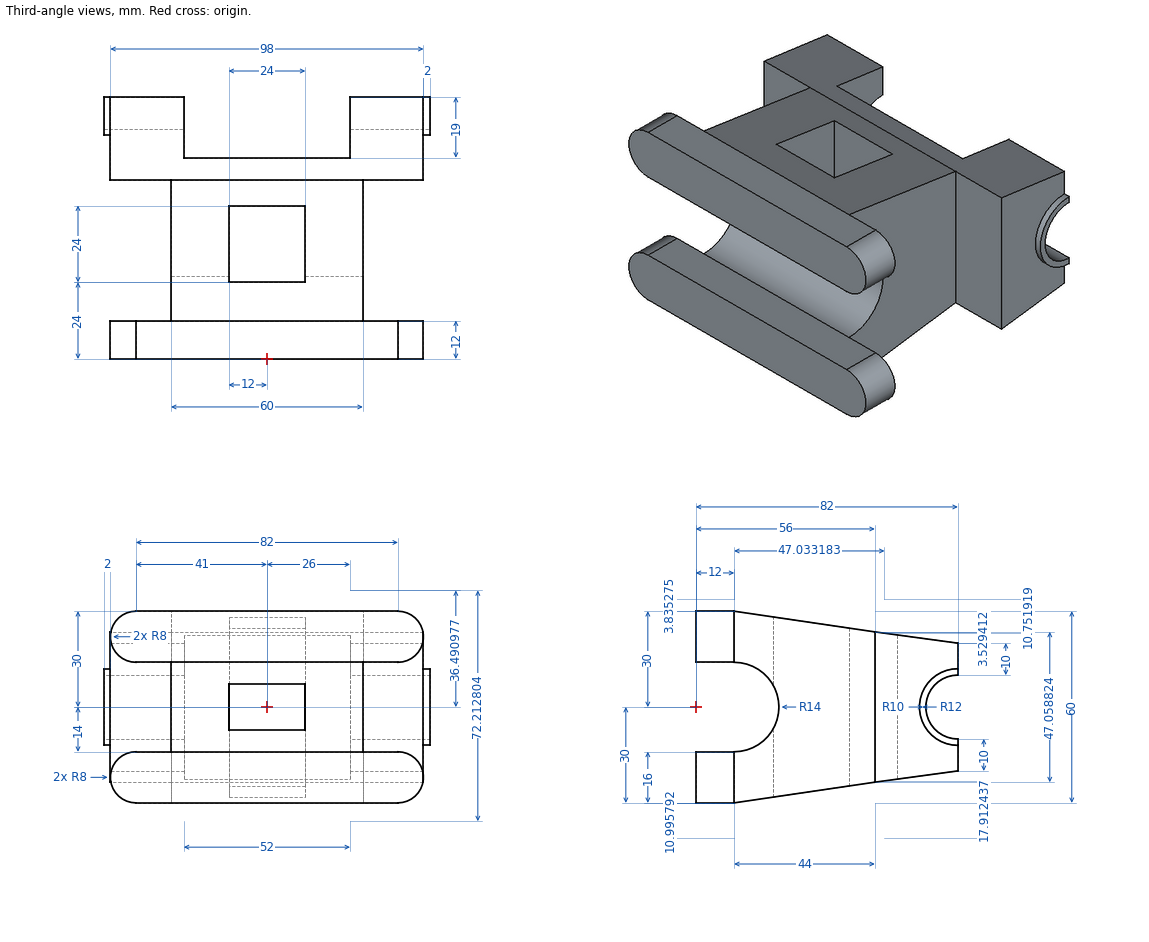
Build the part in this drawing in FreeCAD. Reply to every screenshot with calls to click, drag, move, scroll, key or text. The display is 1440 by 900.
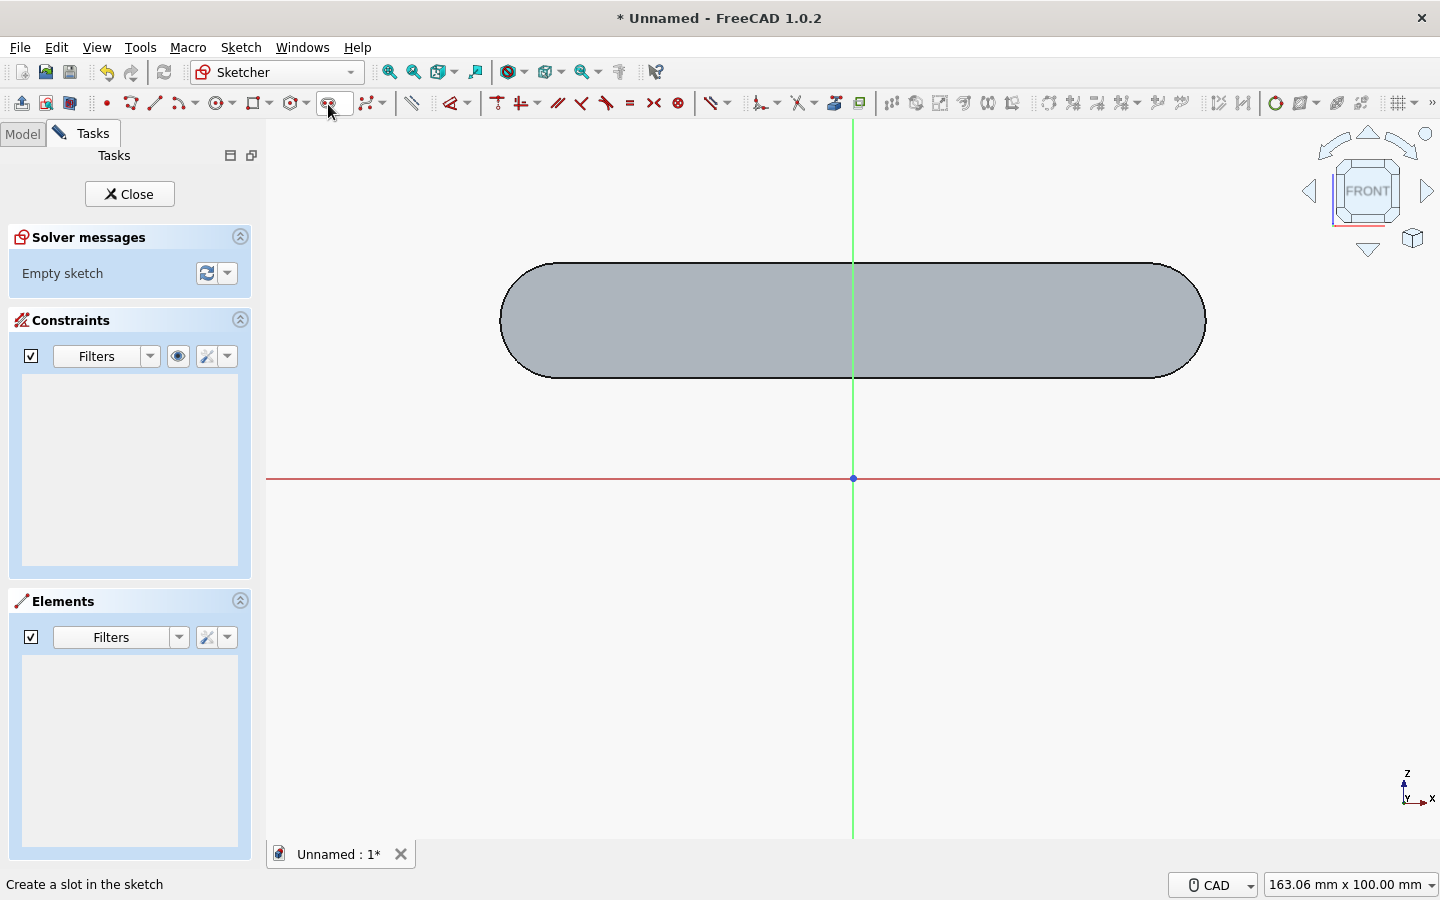
click(558, 637)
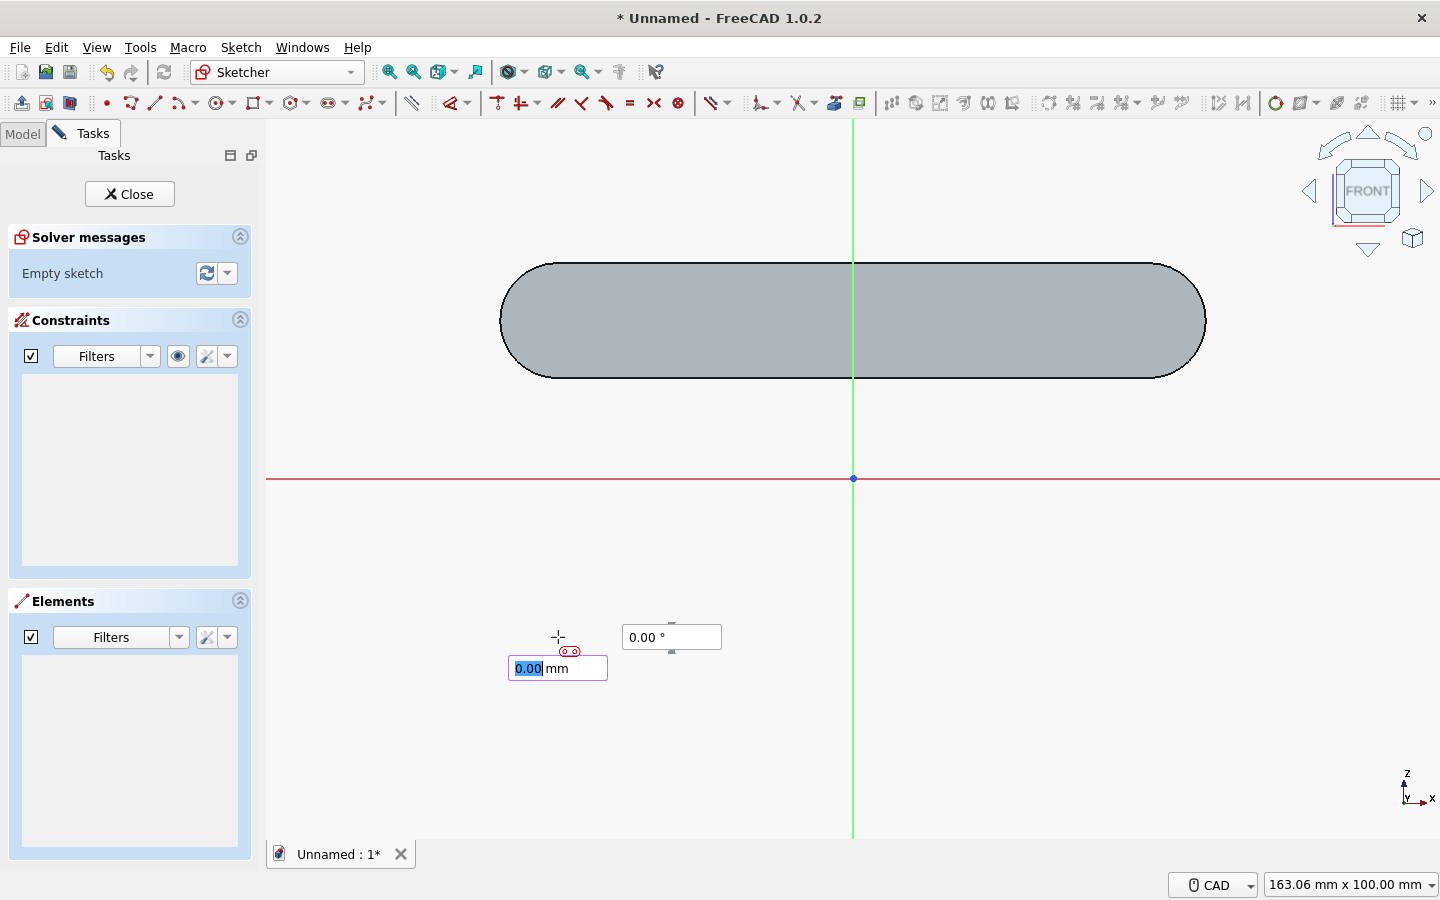
click(1148, 637)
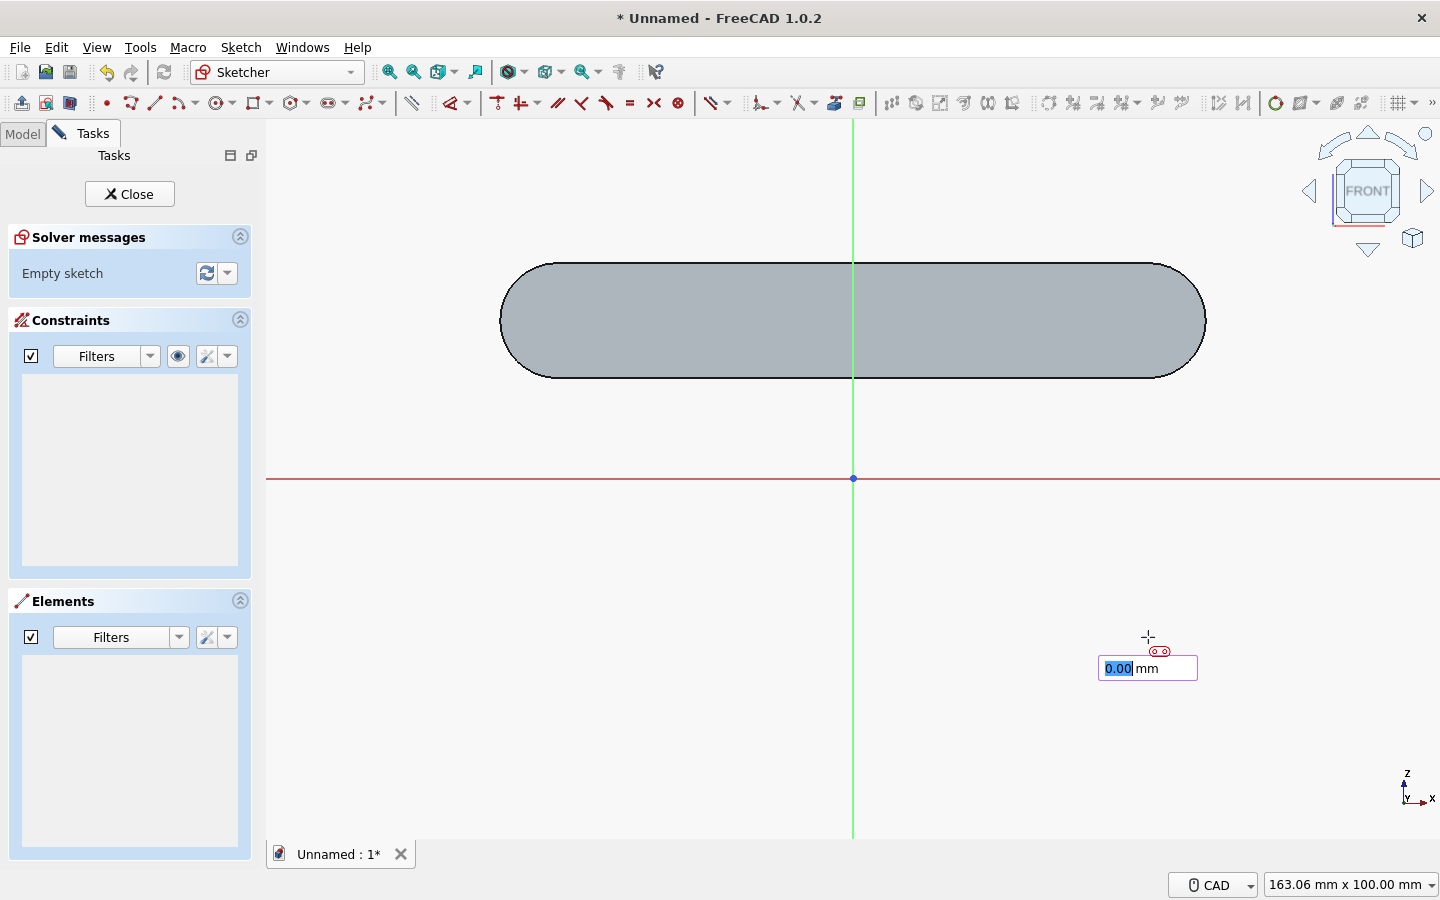
click(942, 695)
key(Escape)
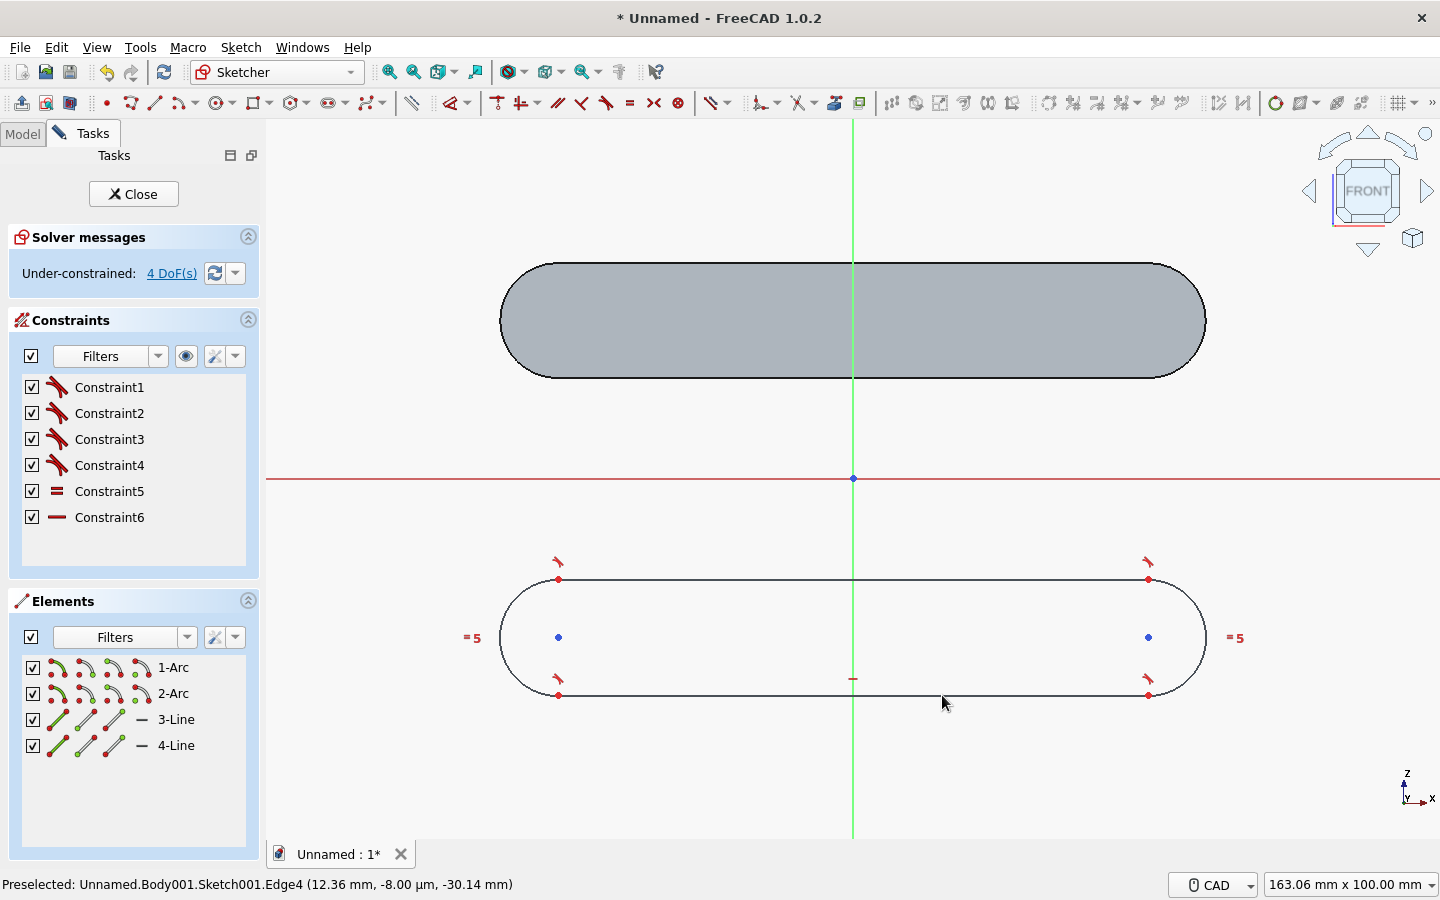
click(450, 104)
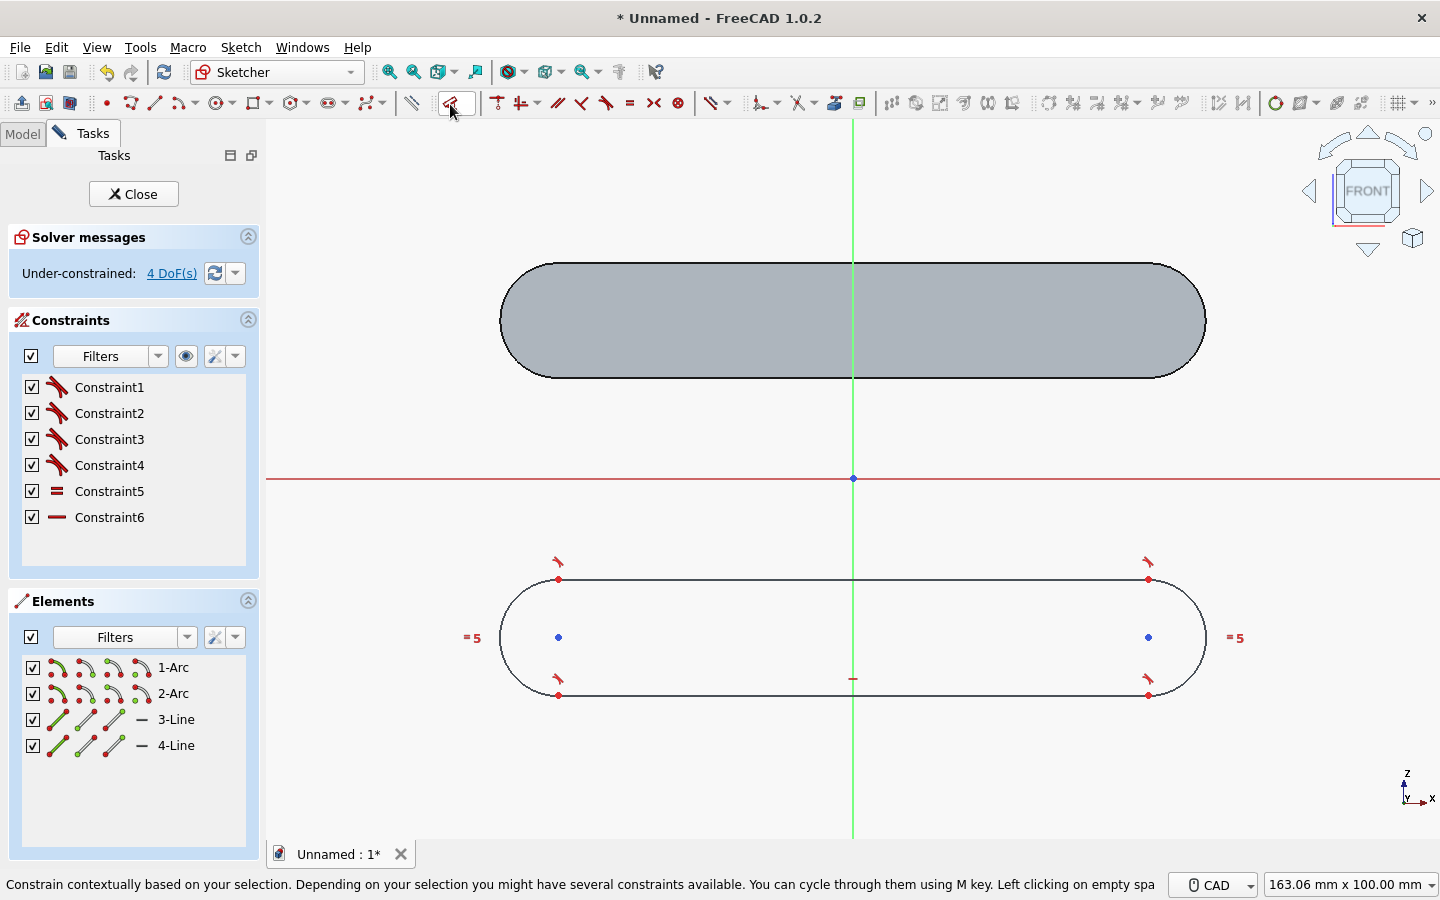
click(511, 604)
click(485, 585)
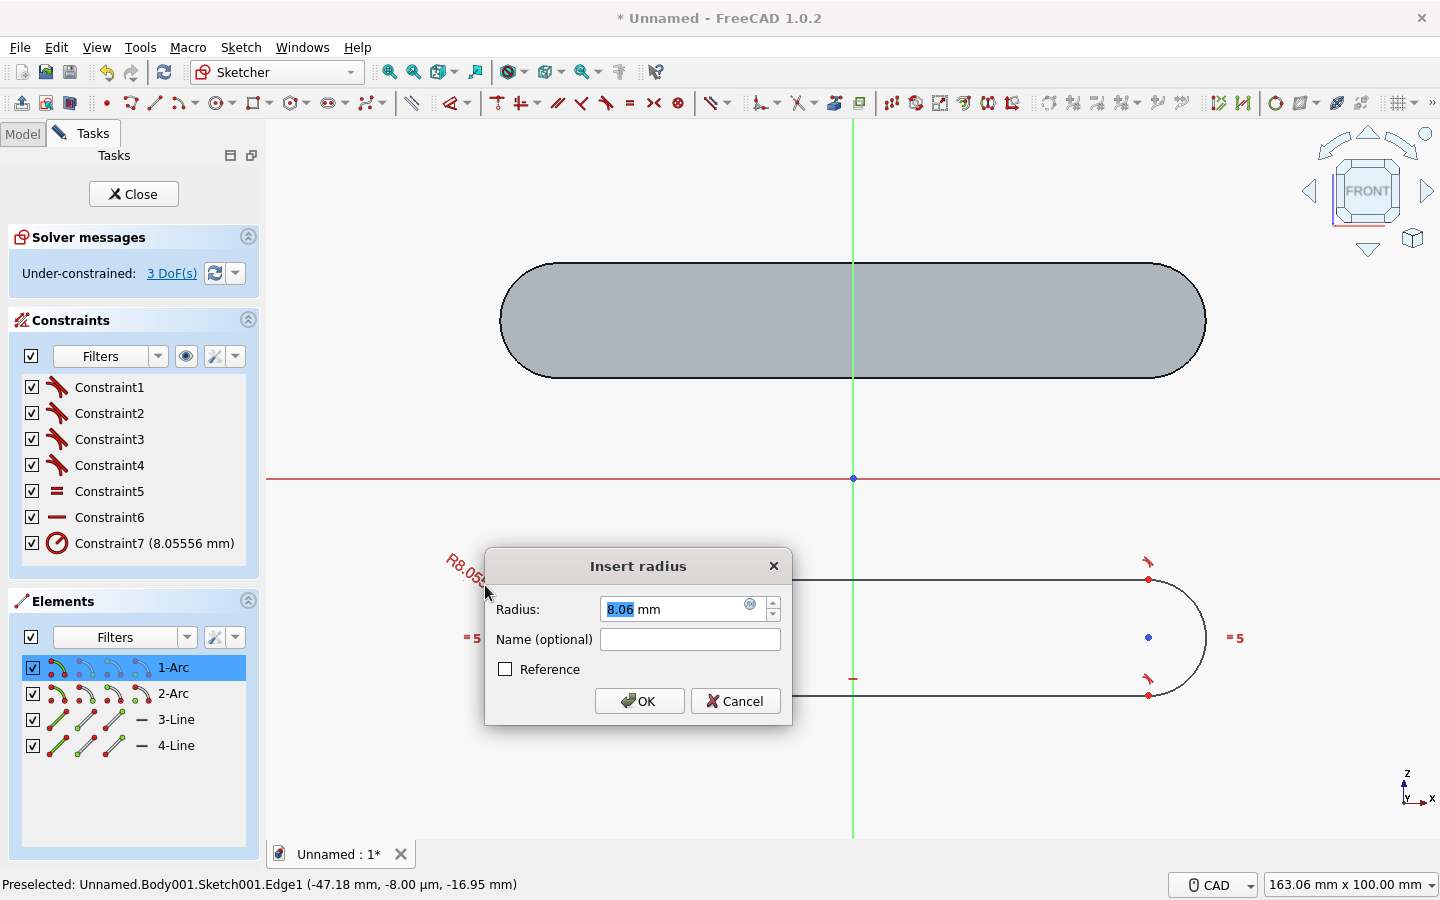
text(8)
key(Return)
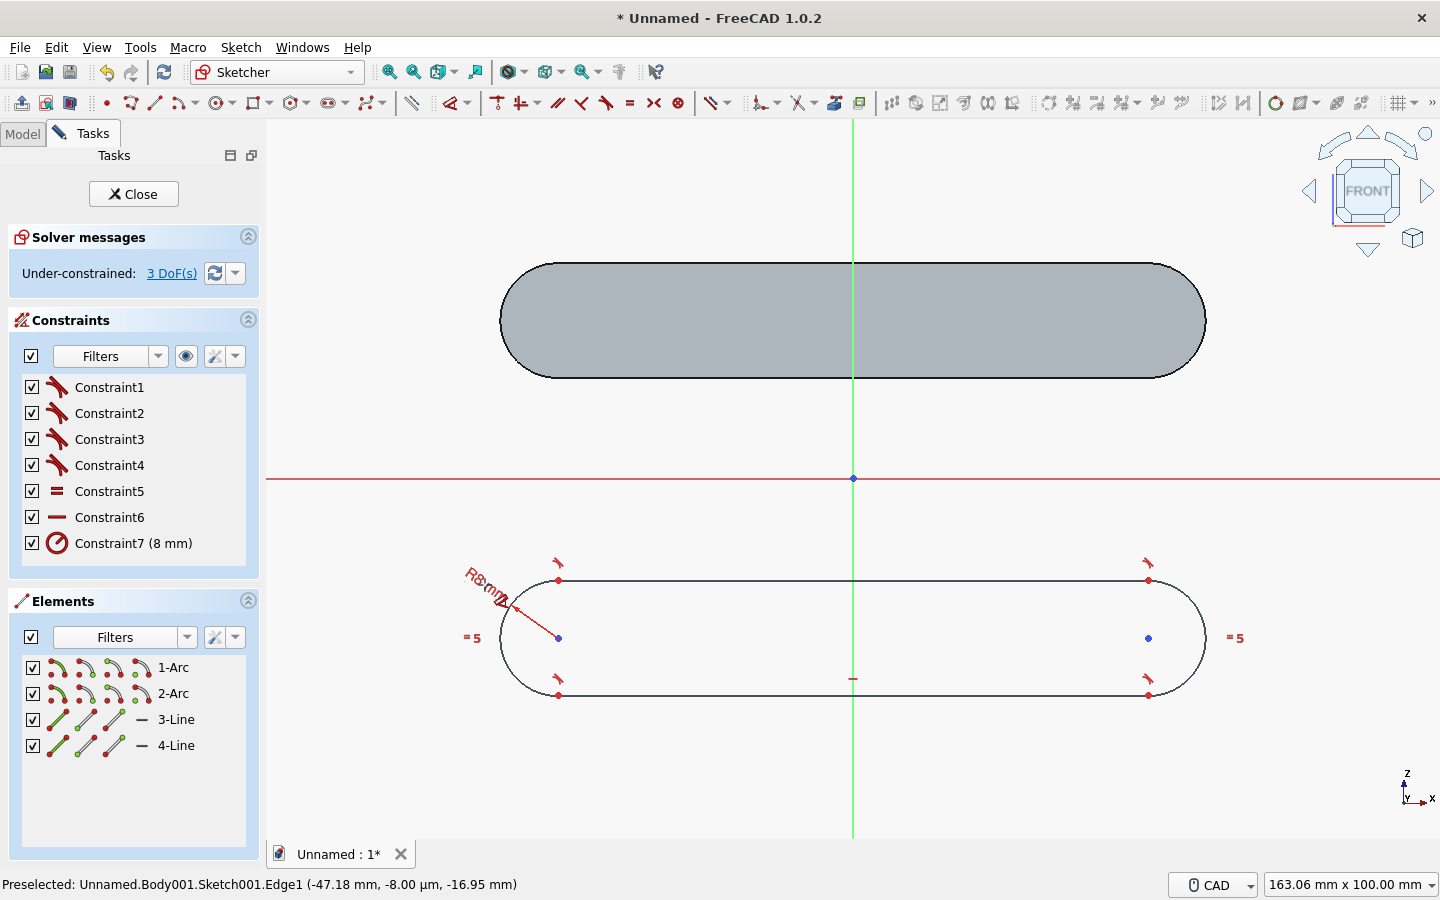
click(735, 581)
click(717, 547)